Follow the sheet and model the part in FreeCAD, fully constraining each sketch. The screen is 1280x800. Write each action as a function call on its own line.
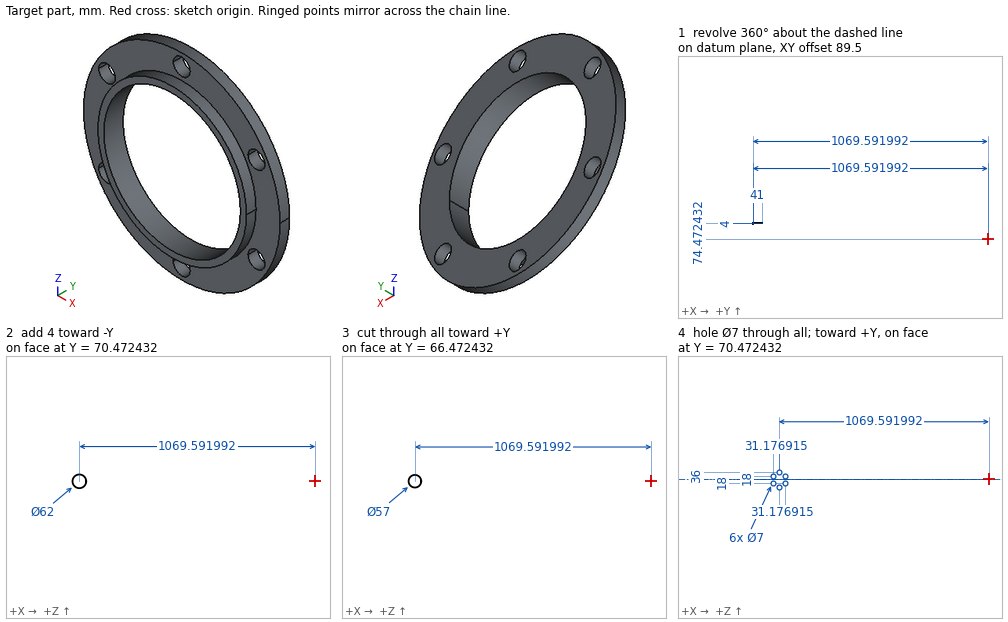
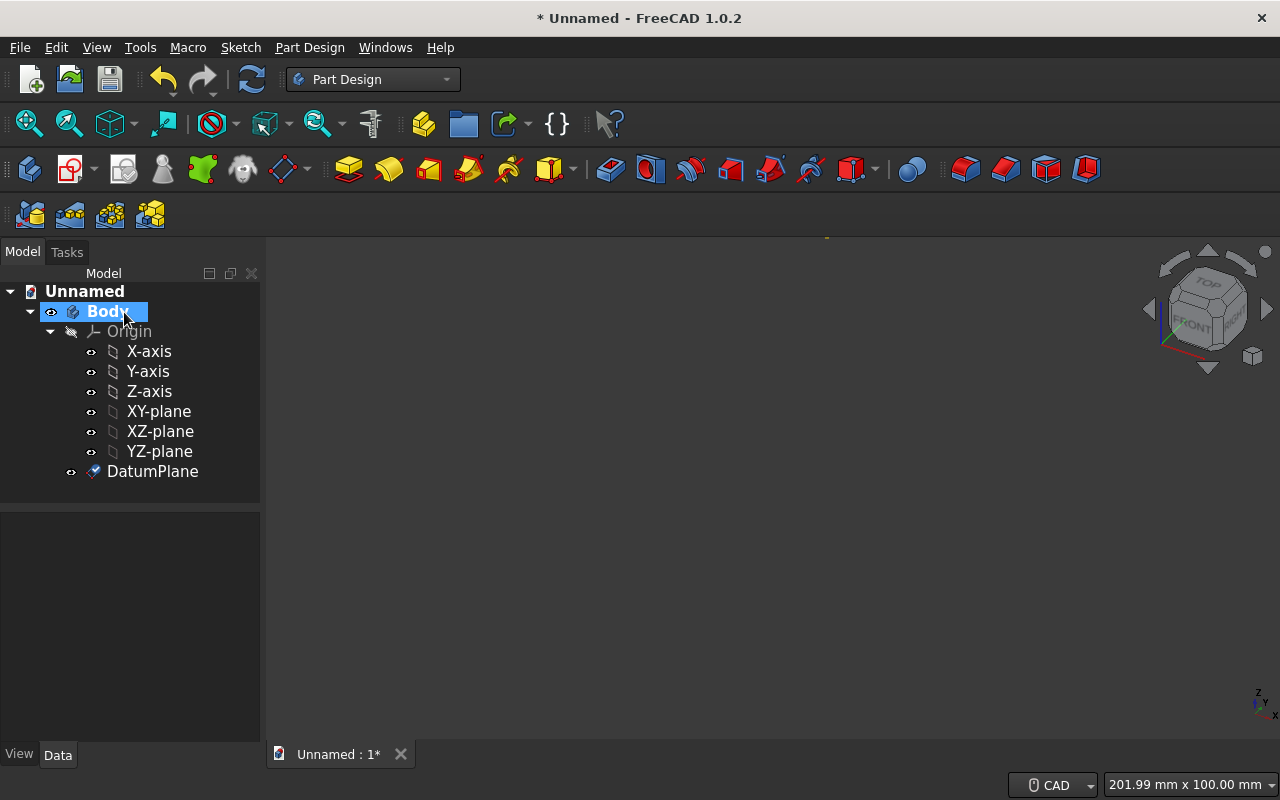
click(116, 472)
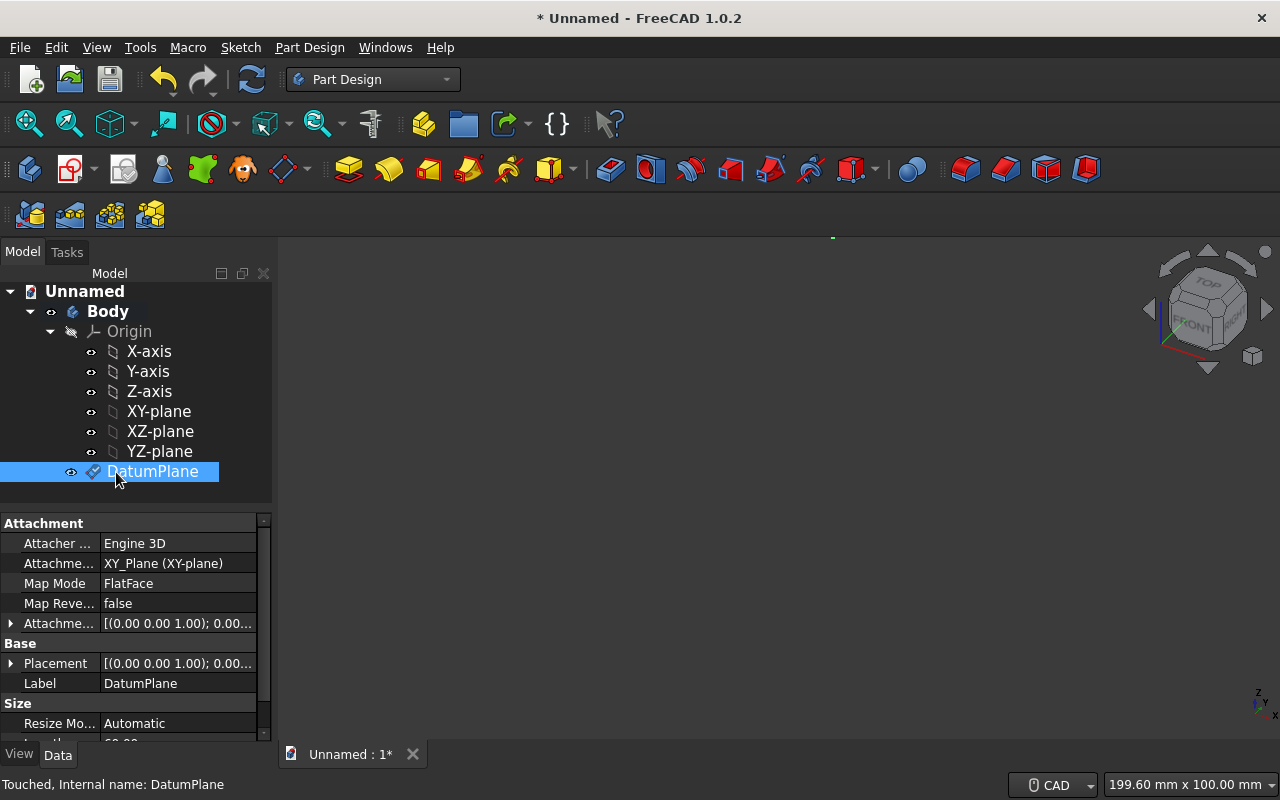
click(70, 170)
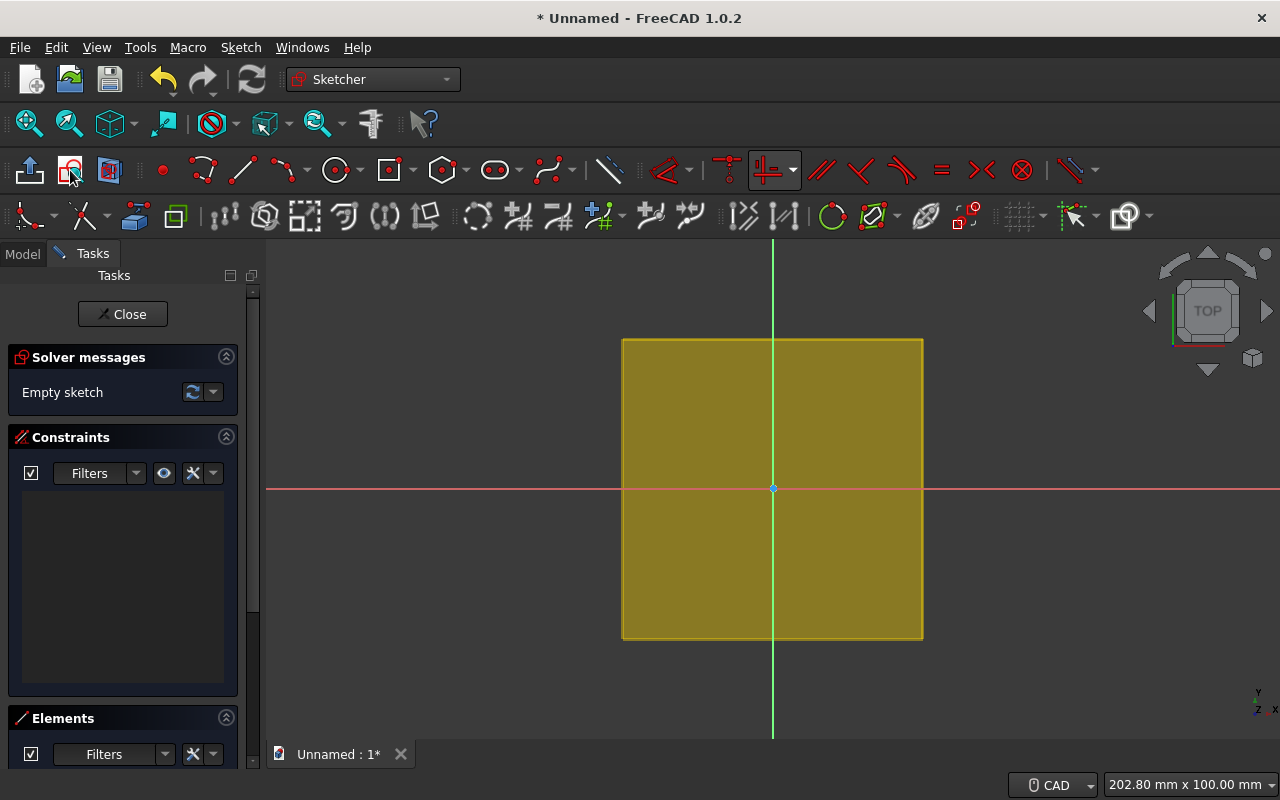
scroll(704, 489, down, 5)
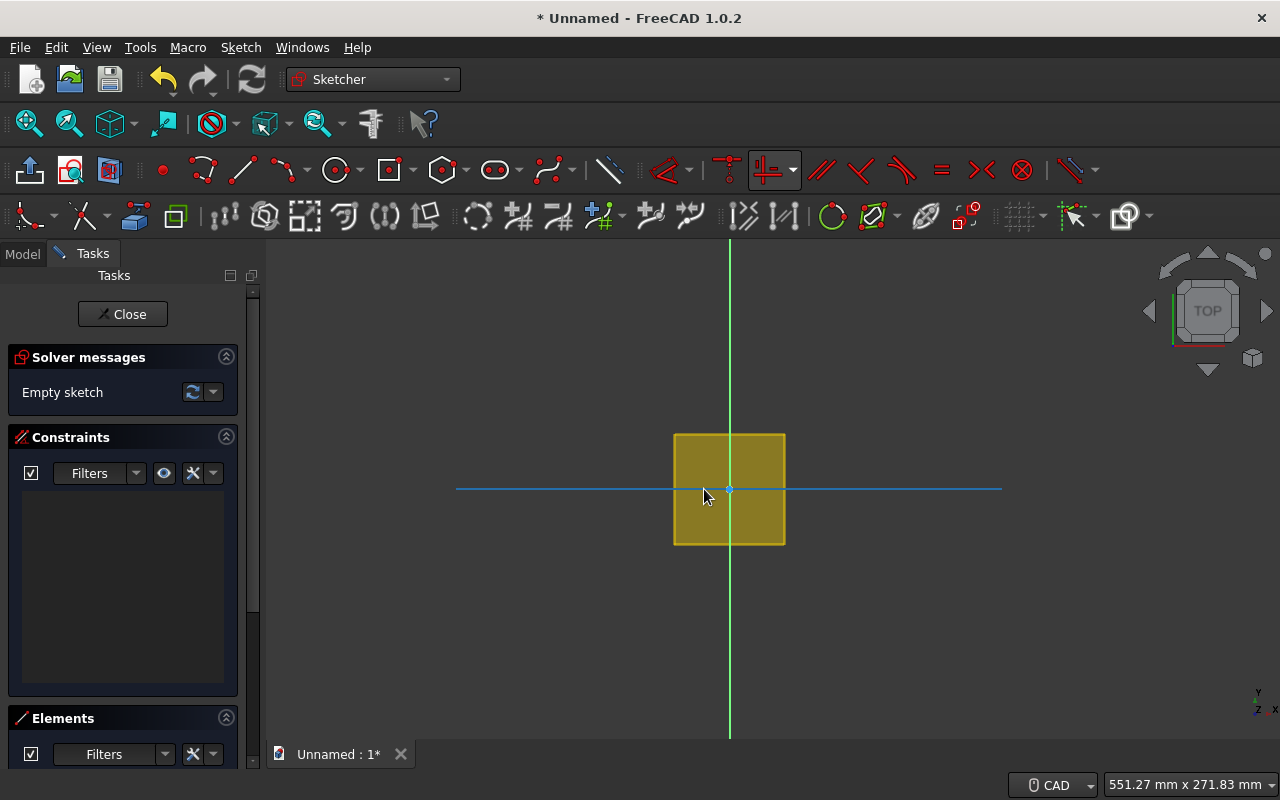
scroll(704, 489, down, 5)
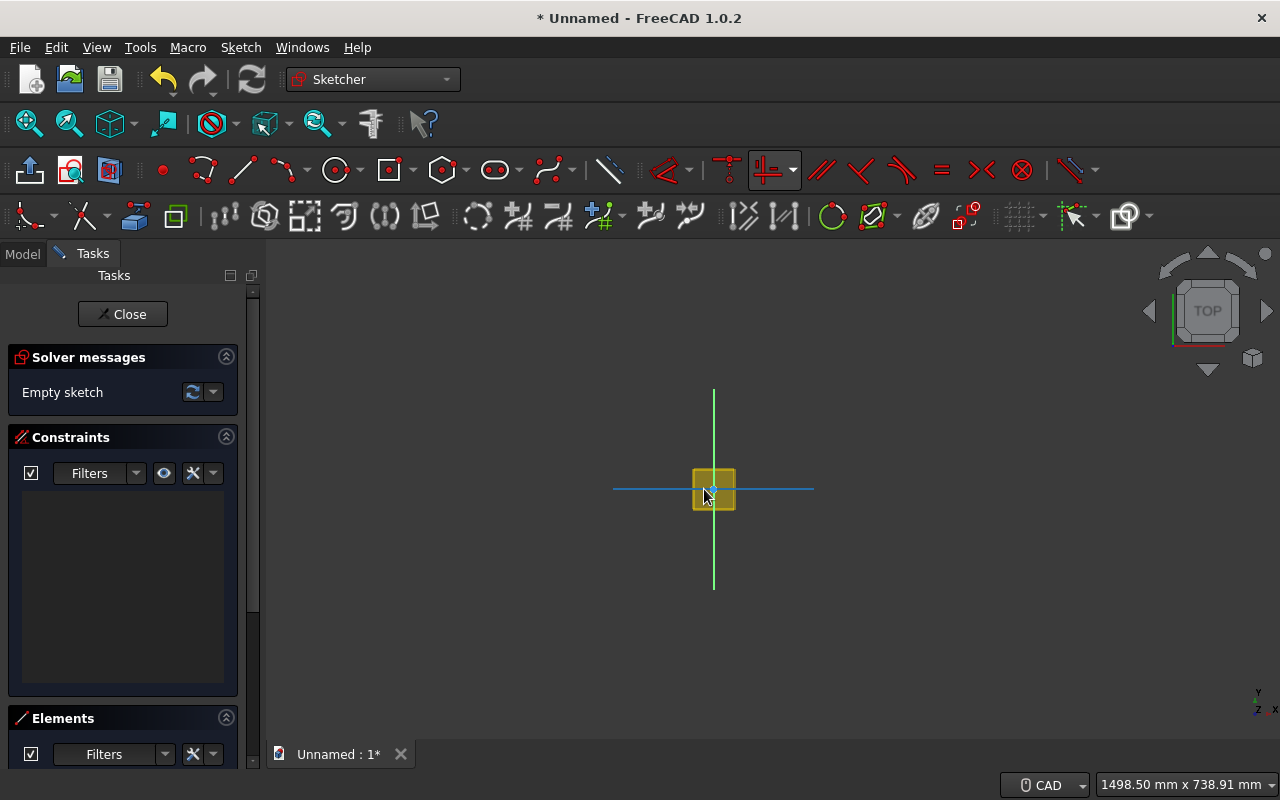
scroll(704, 489, down, 5)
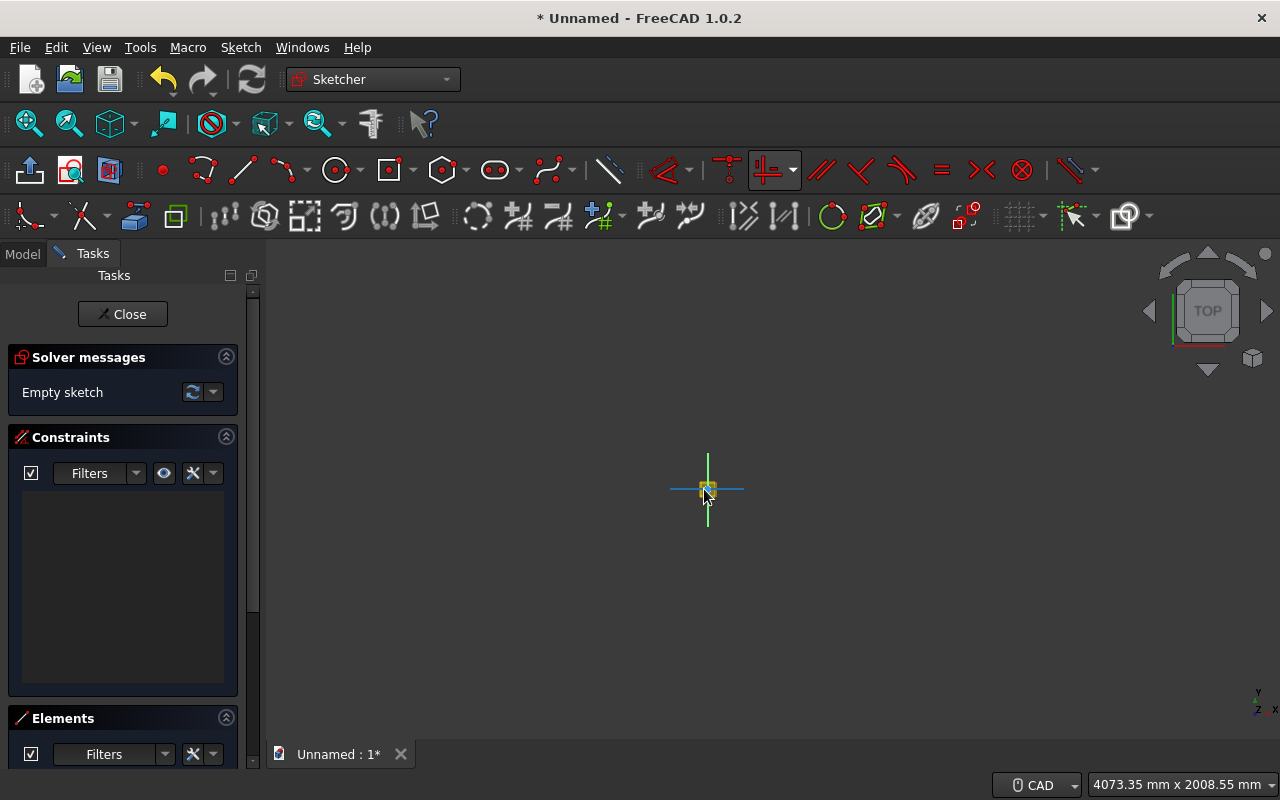
scroll(433, 471, up, 15)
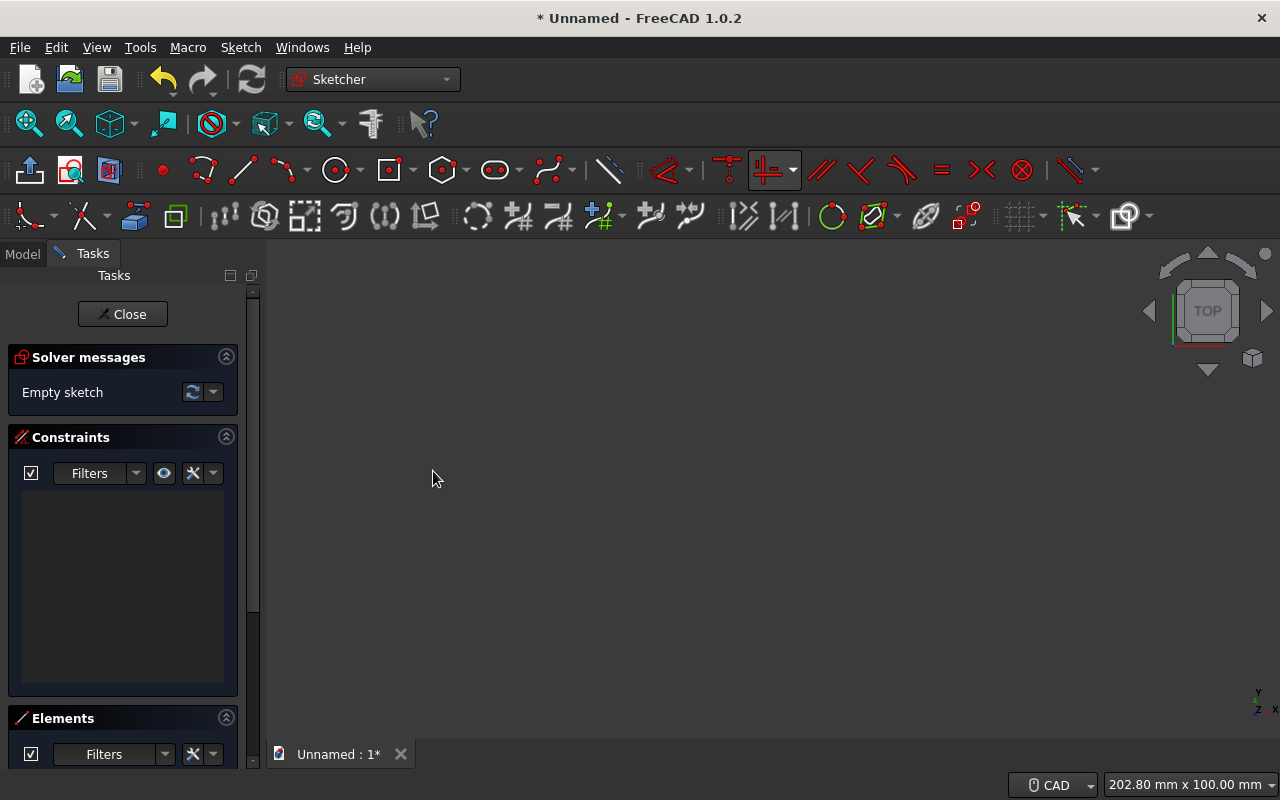
scroll(705, 486, up, 5)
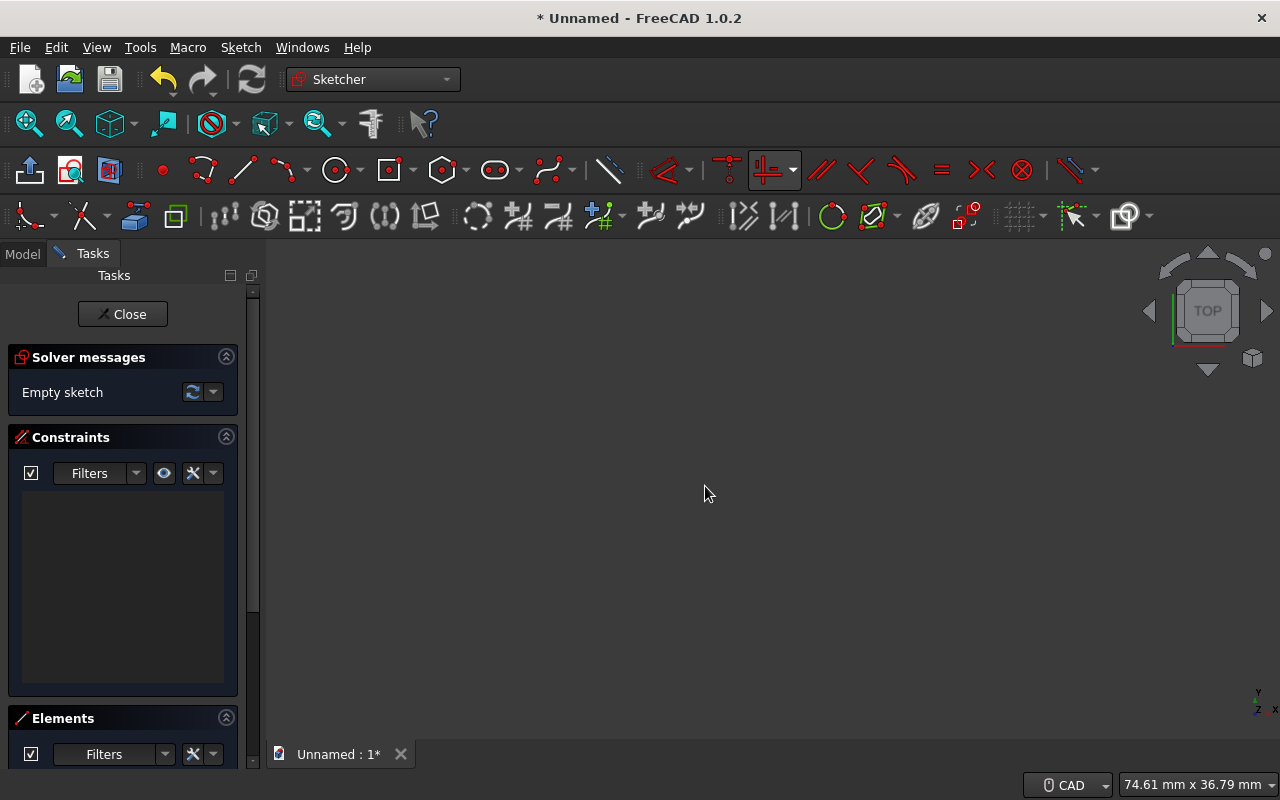
key(g)
key(r)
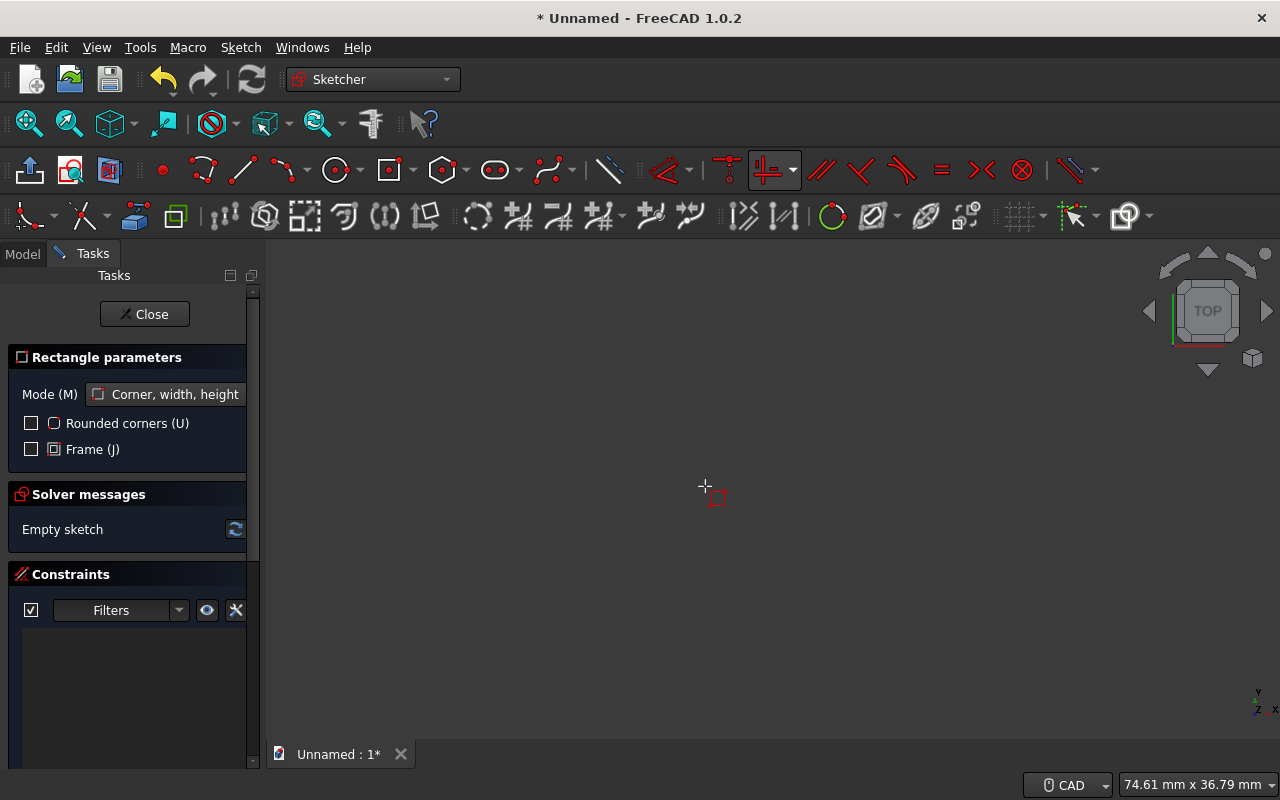
click(425, 417)
move(982, 471)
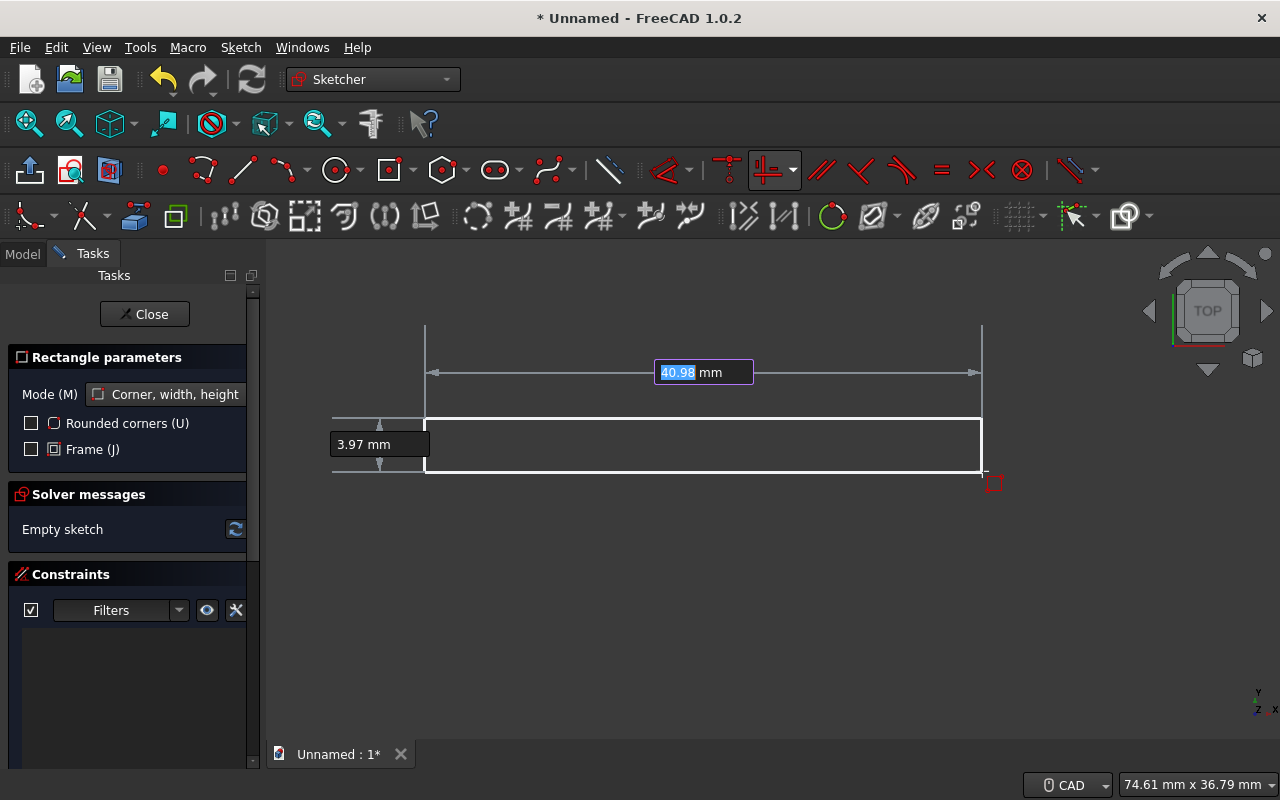
text(41)
key(Tab)
text(4)
key(Return)